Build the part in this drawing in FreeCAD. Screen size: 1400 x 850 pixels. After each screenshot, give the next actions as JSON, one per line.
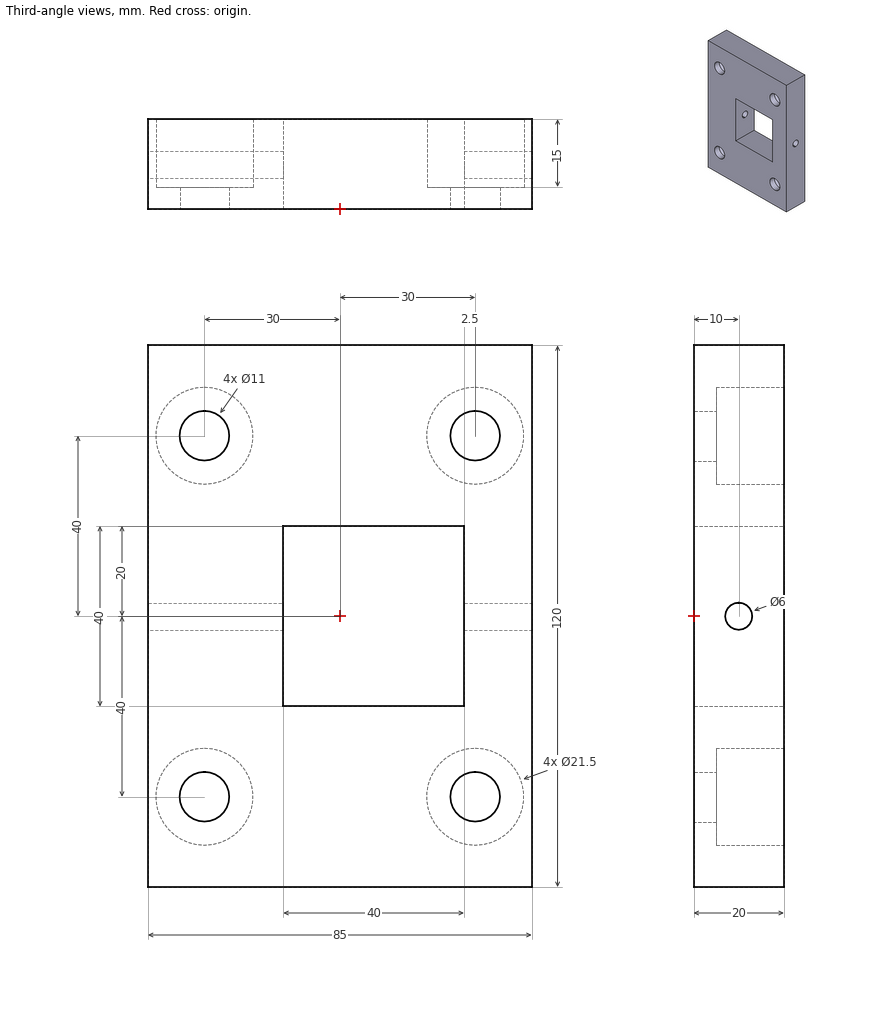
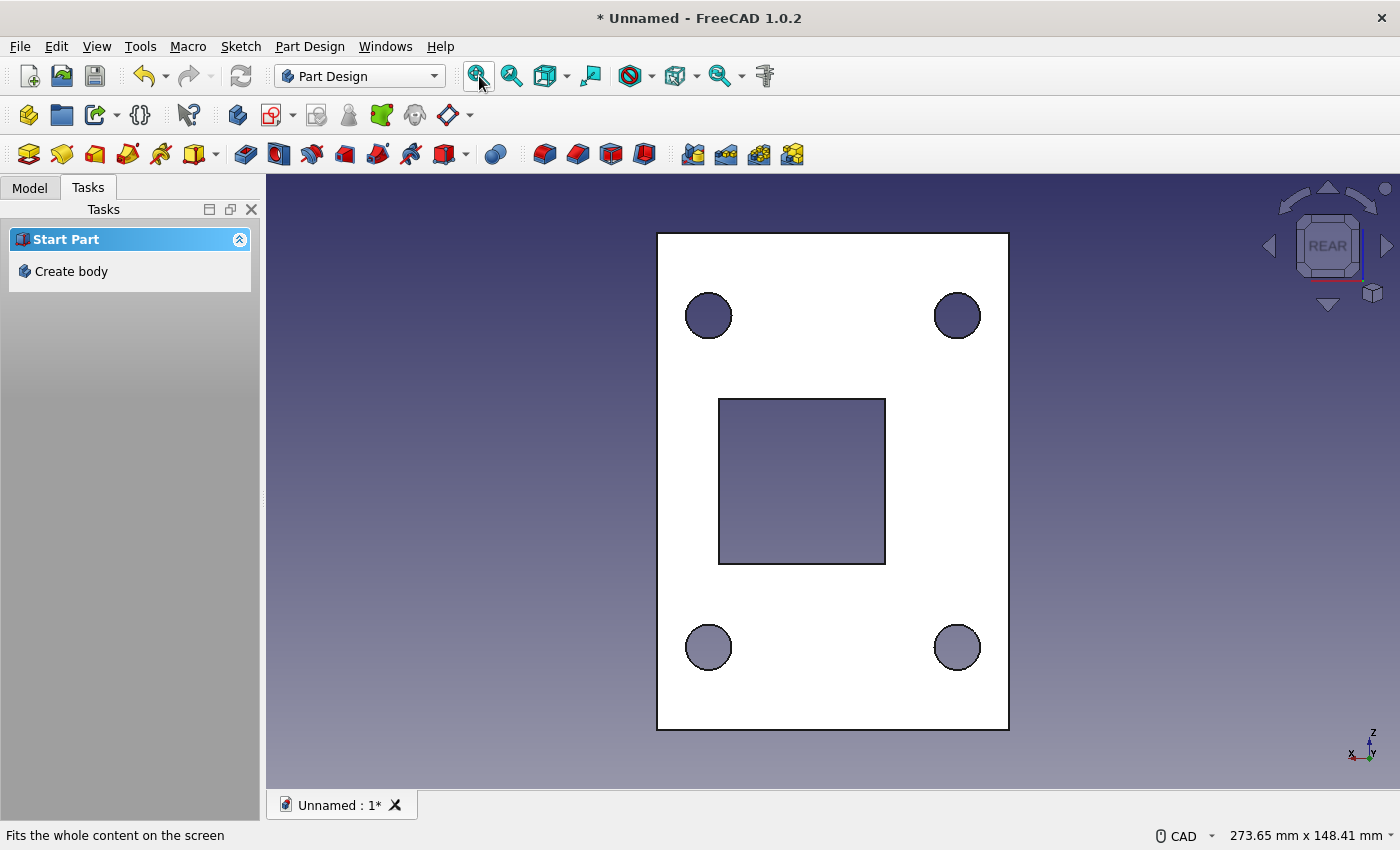
{"action": "left_click", "coordinate": [833, 338]}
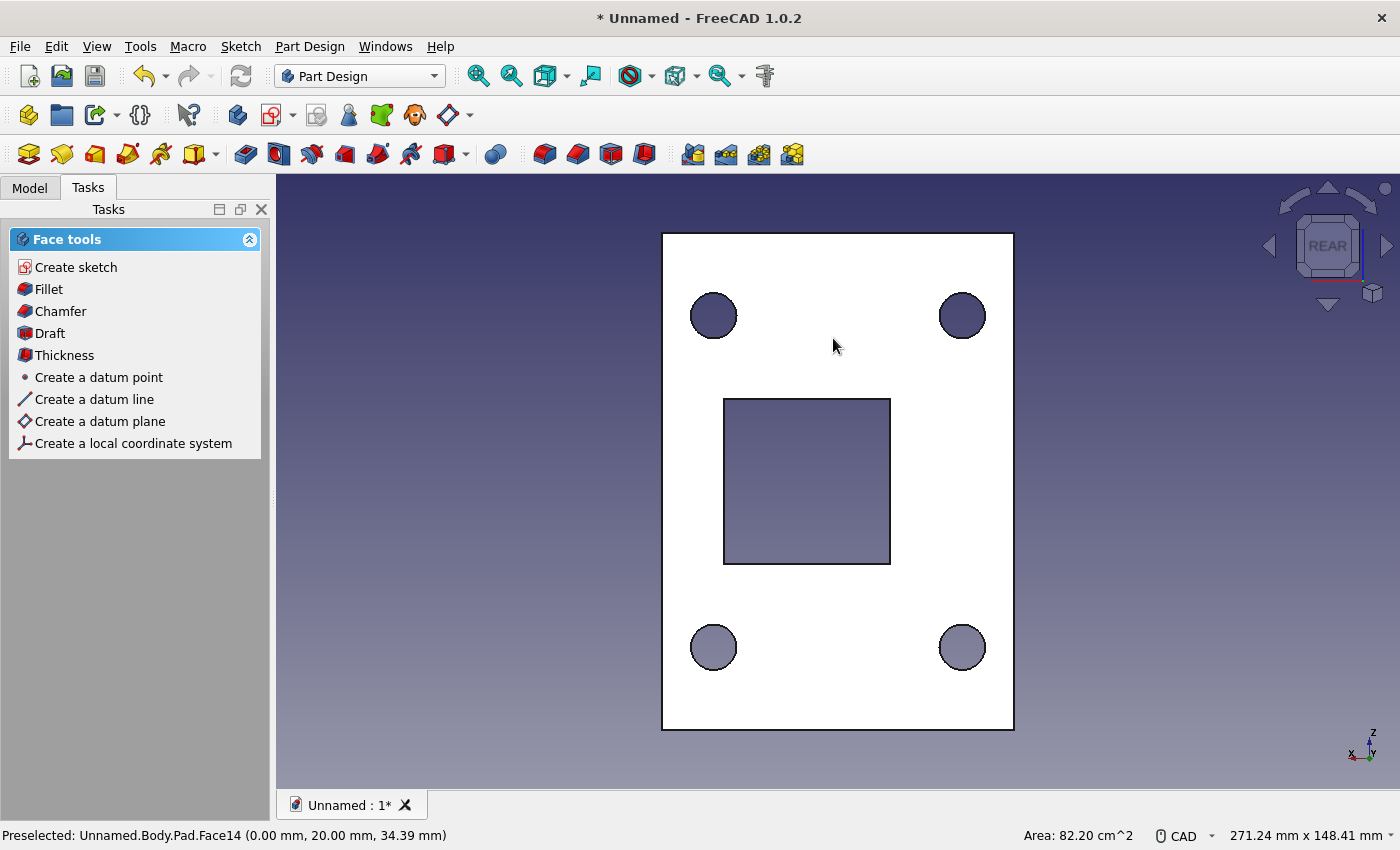
{"action": "left_click", "coordinate": [270, 116]}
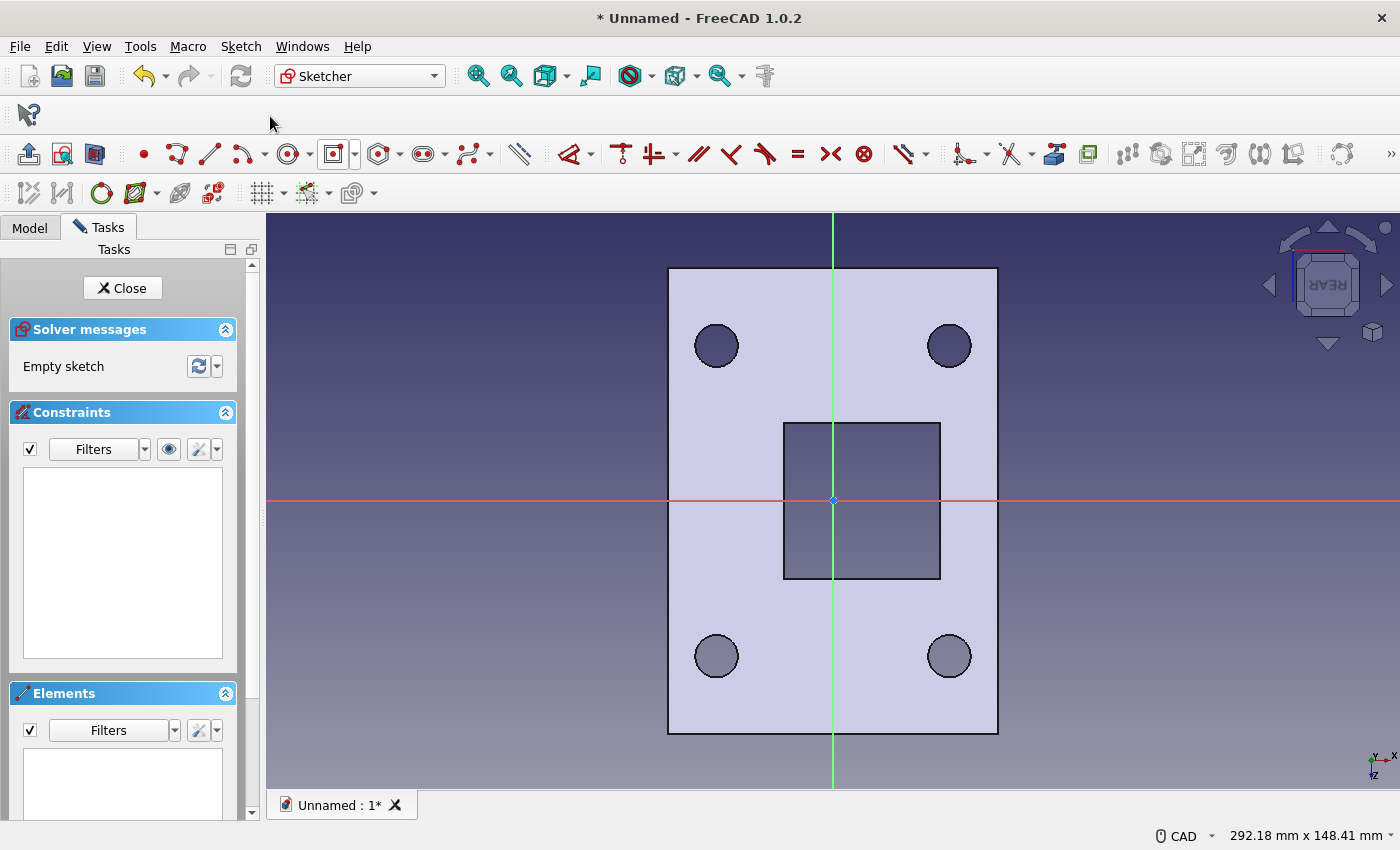
{"action": "key", "text": "g c"}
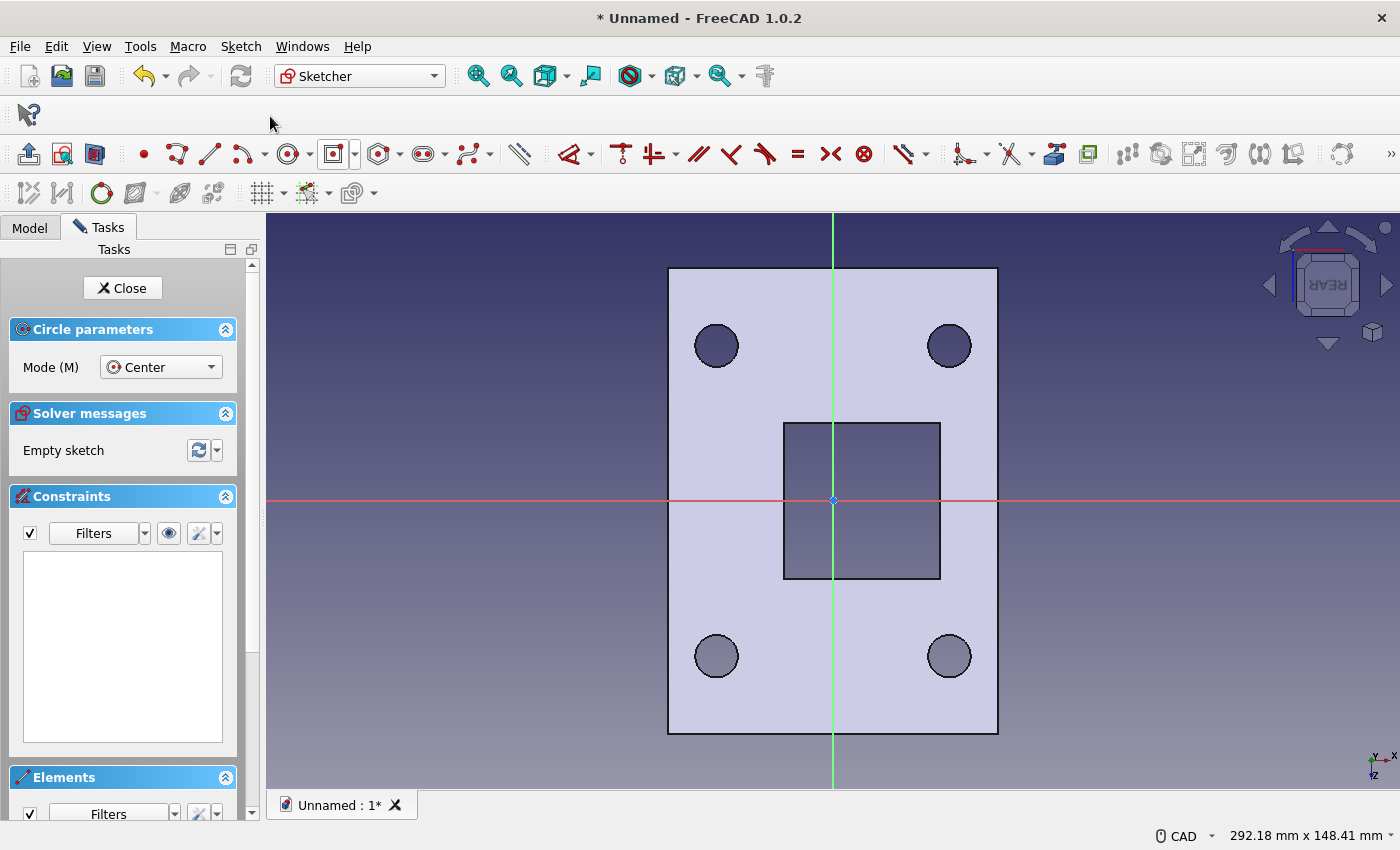
{"action": "left_click", "coordinate": [949, 346]}
{"action": "left_click", "coordinate": [979, 316]}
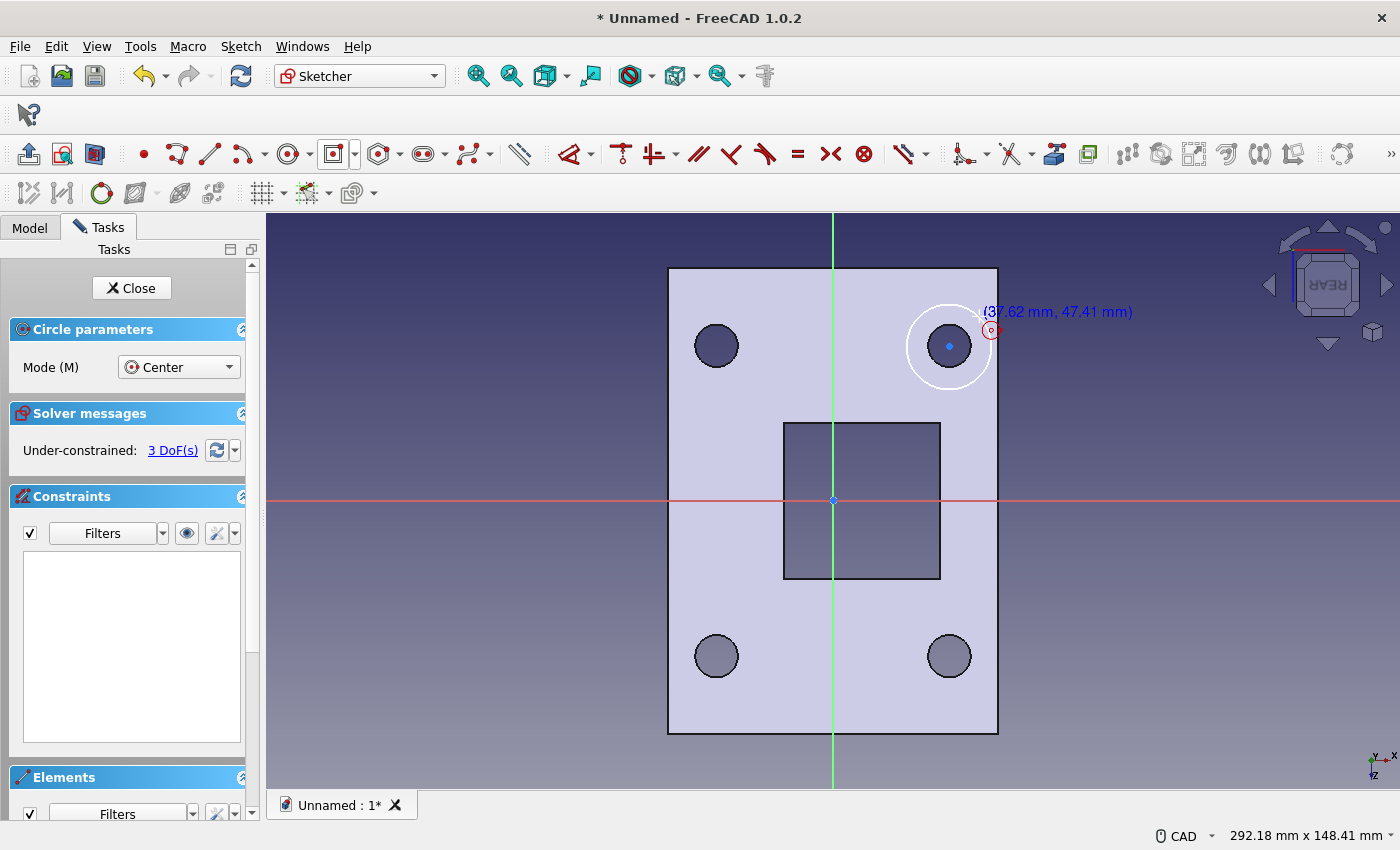
{"action": "left_click", "coordinate": [717, 346]}
{"action": "left_click", "coordinate": [746, 316]}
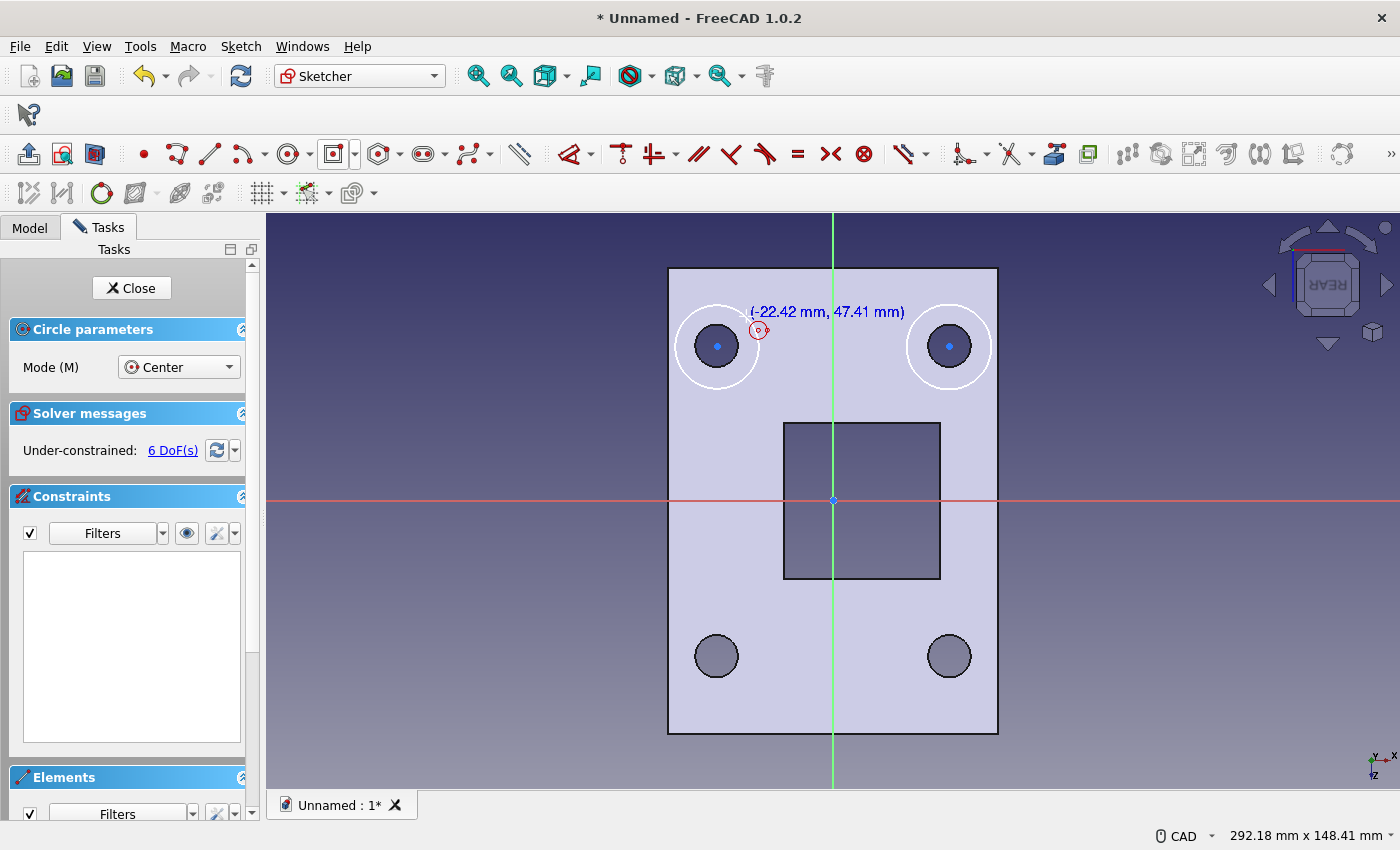
{"action": "left_click", "coordinate": [717, 656]}
{"action": "left_click", "coordinate": [746, 627]}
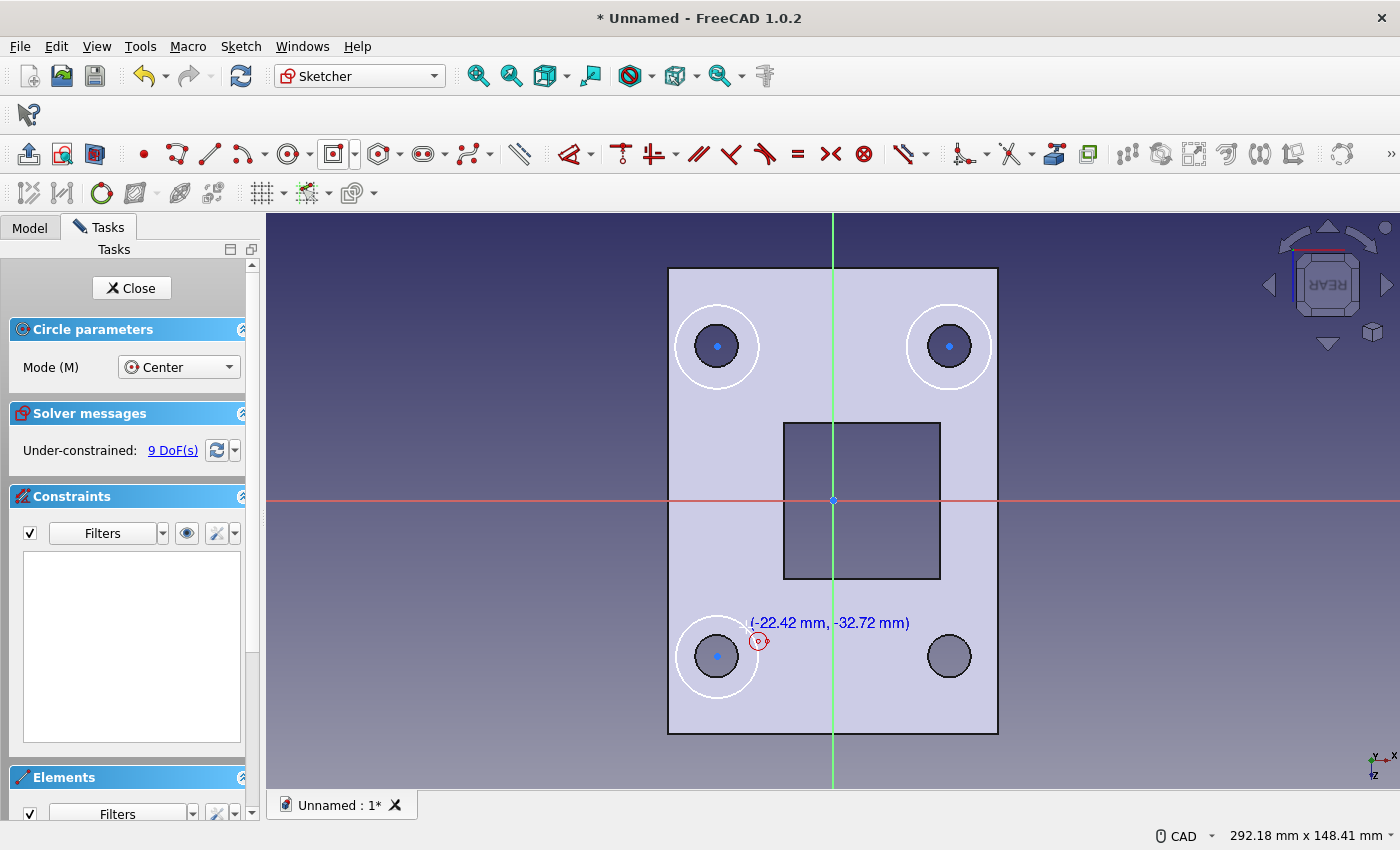
{"action": "left_click", "coordinate": [949, 656]}
{"action": "left_click", "coordinate": [979, 627]}
{"action": "key", "text": "Escape"}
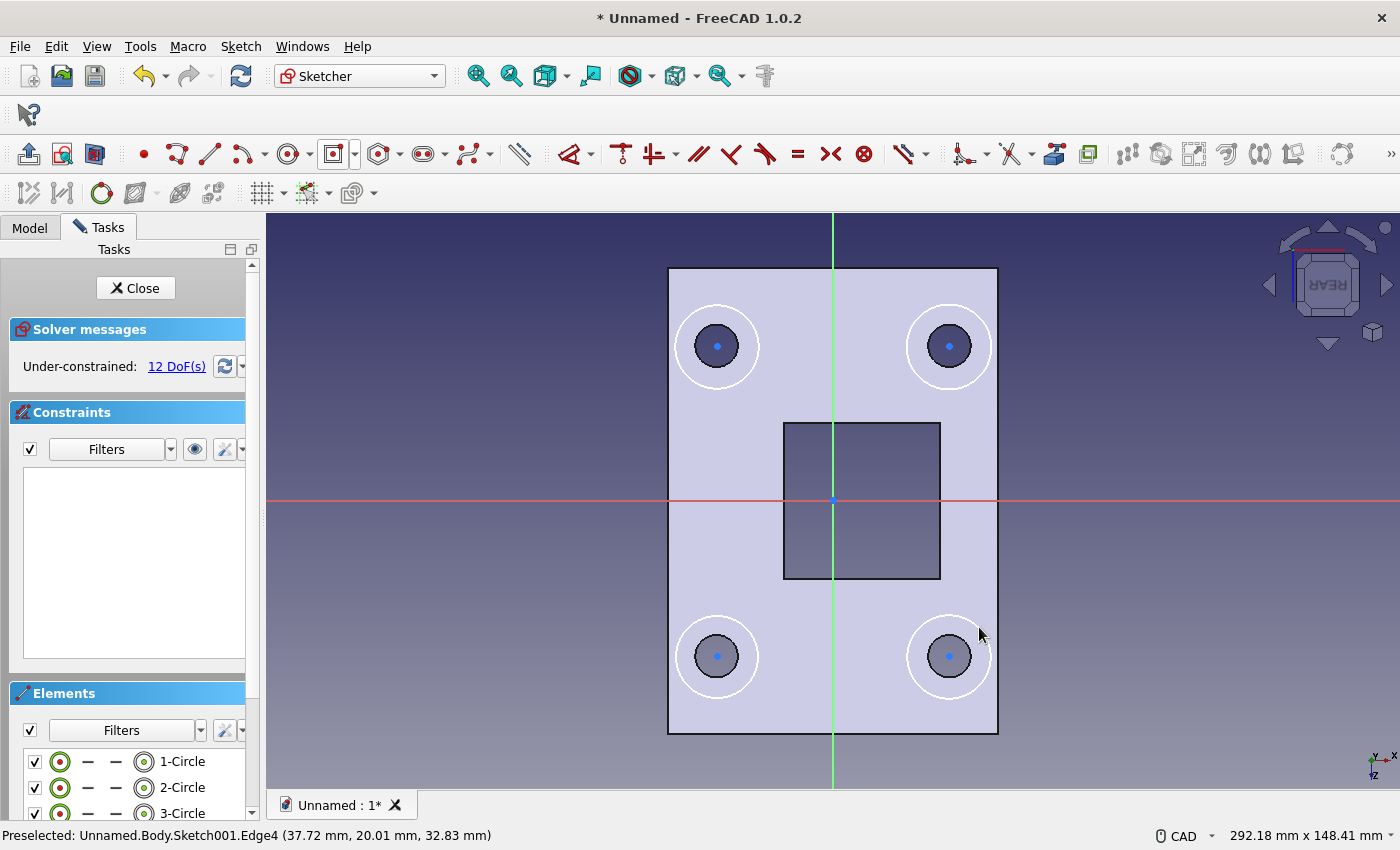
{"action": "left_click", "coordinate": [979, 317]}